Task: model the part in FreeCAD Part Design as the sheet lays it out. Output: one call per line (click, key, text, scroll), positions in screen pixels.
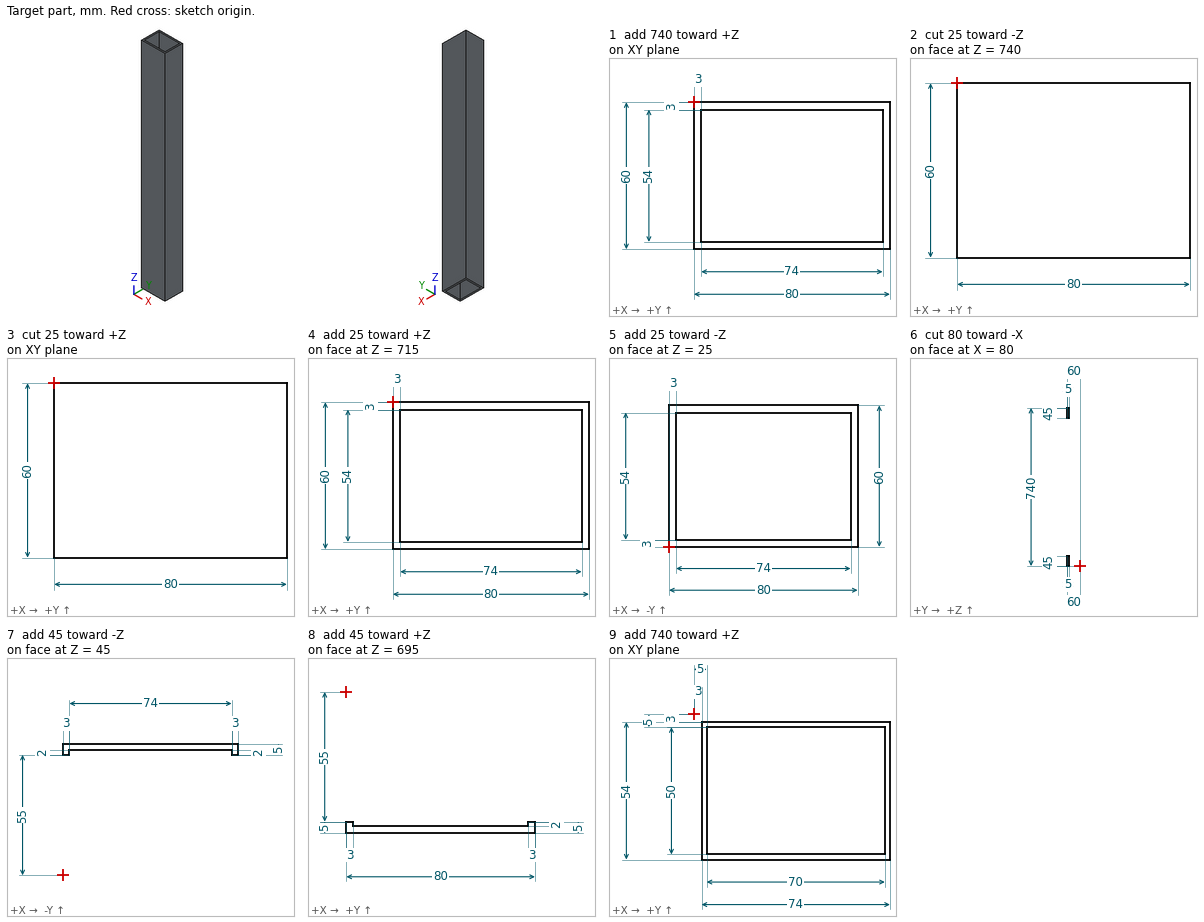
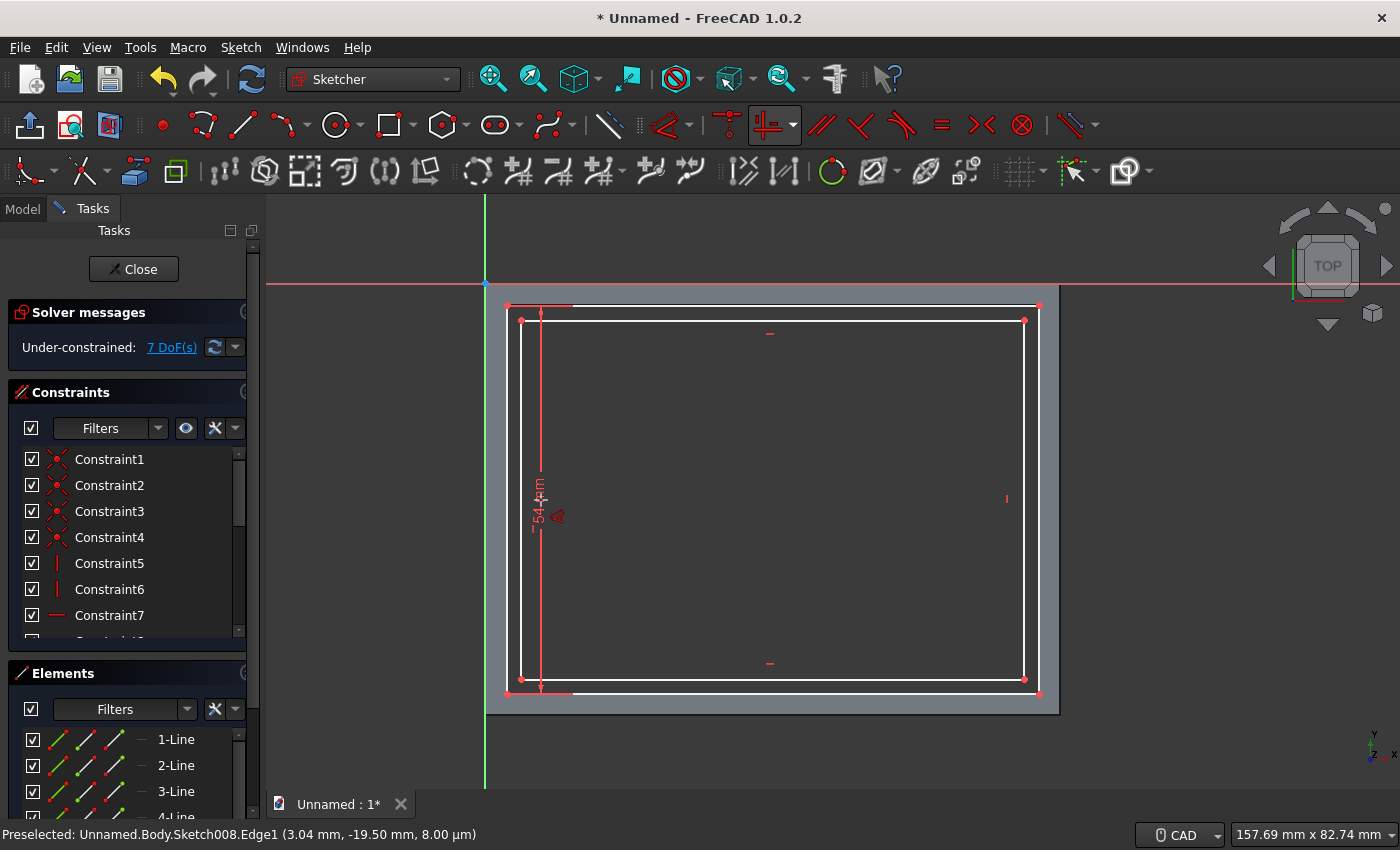
click(667, 694)
click(773, 728)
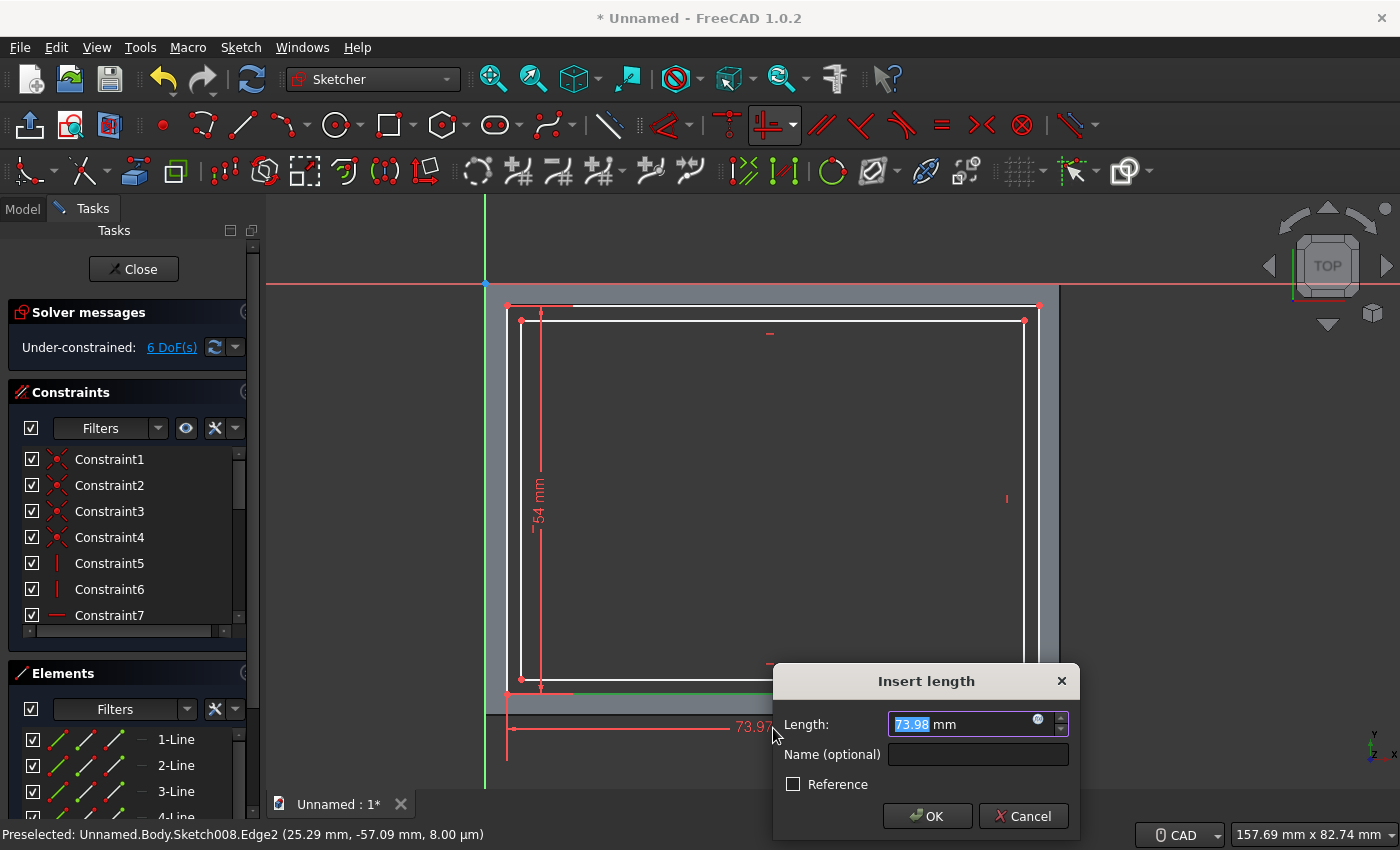
text(74)
key(Return)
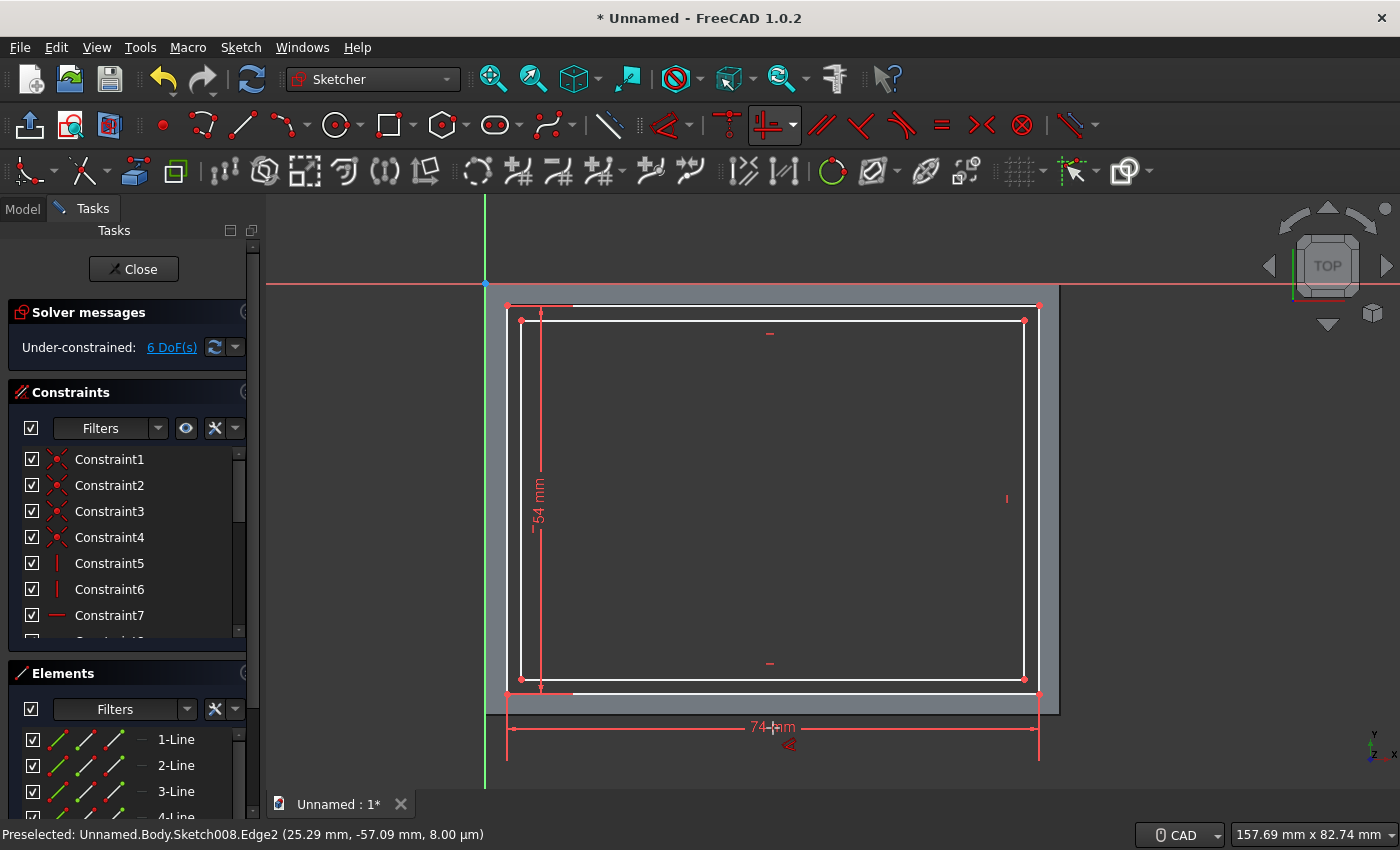
click(521, 429)
click(555, 418)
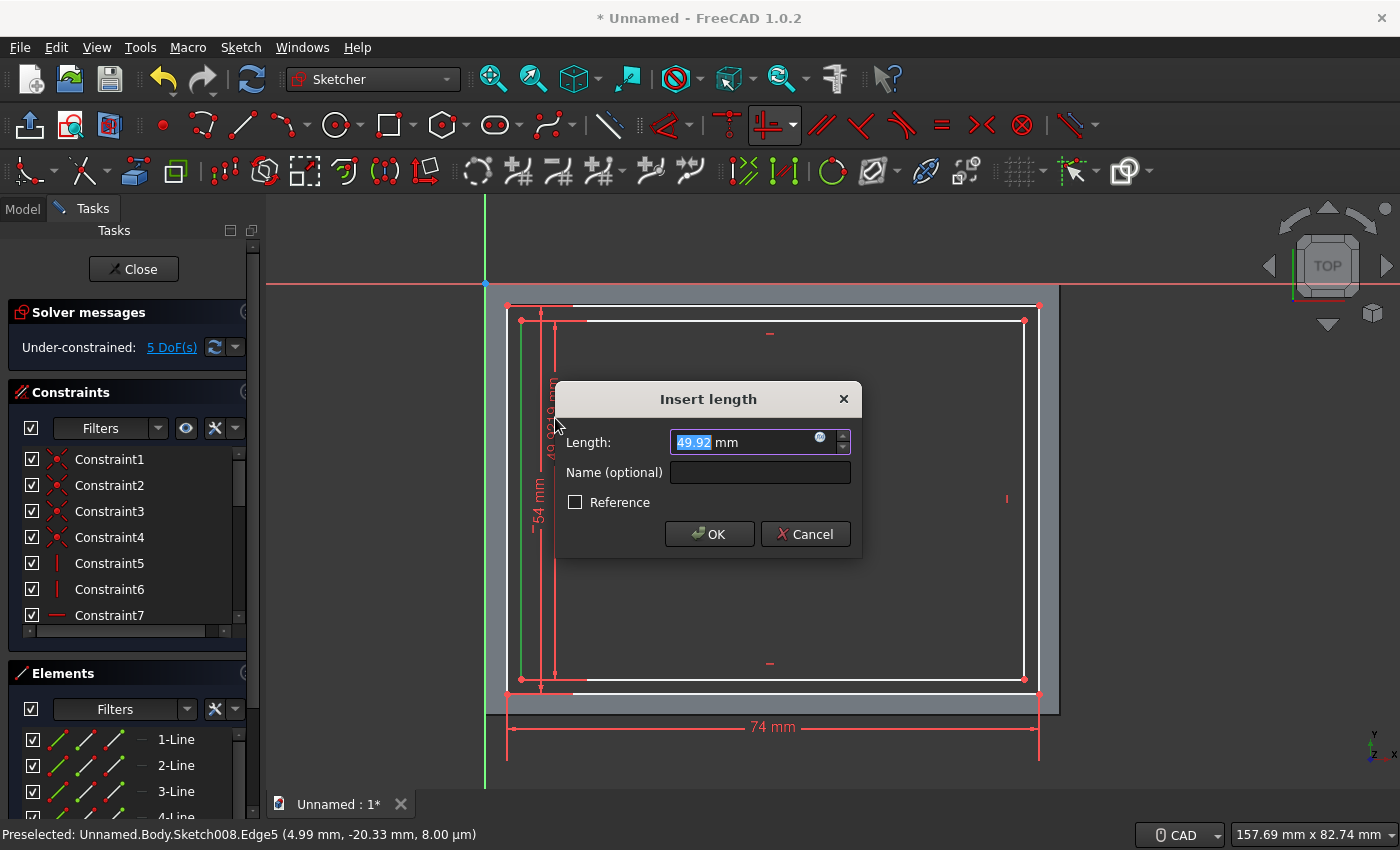
text(50)
key(Return)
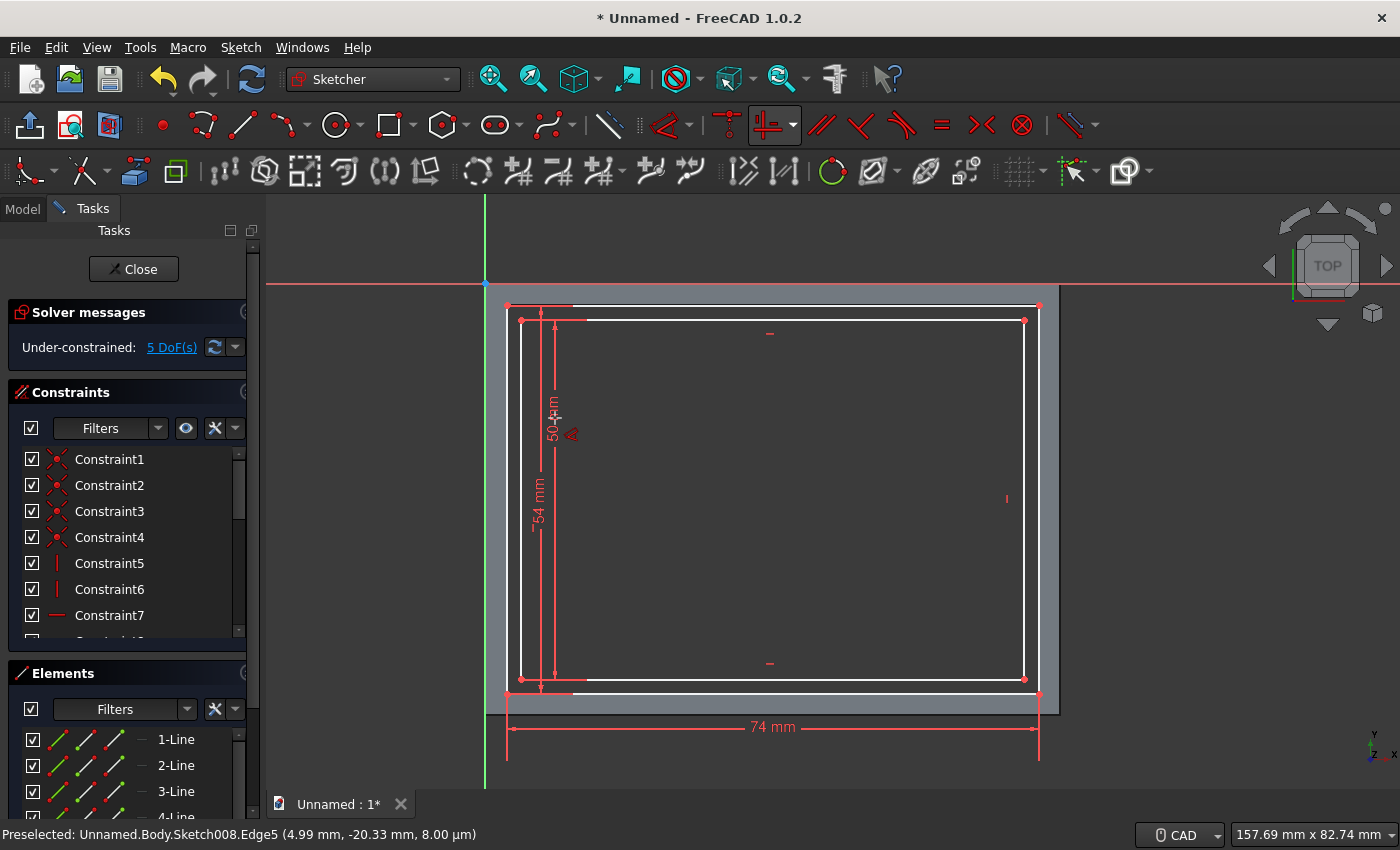
click(672, 680)
click(657, 714)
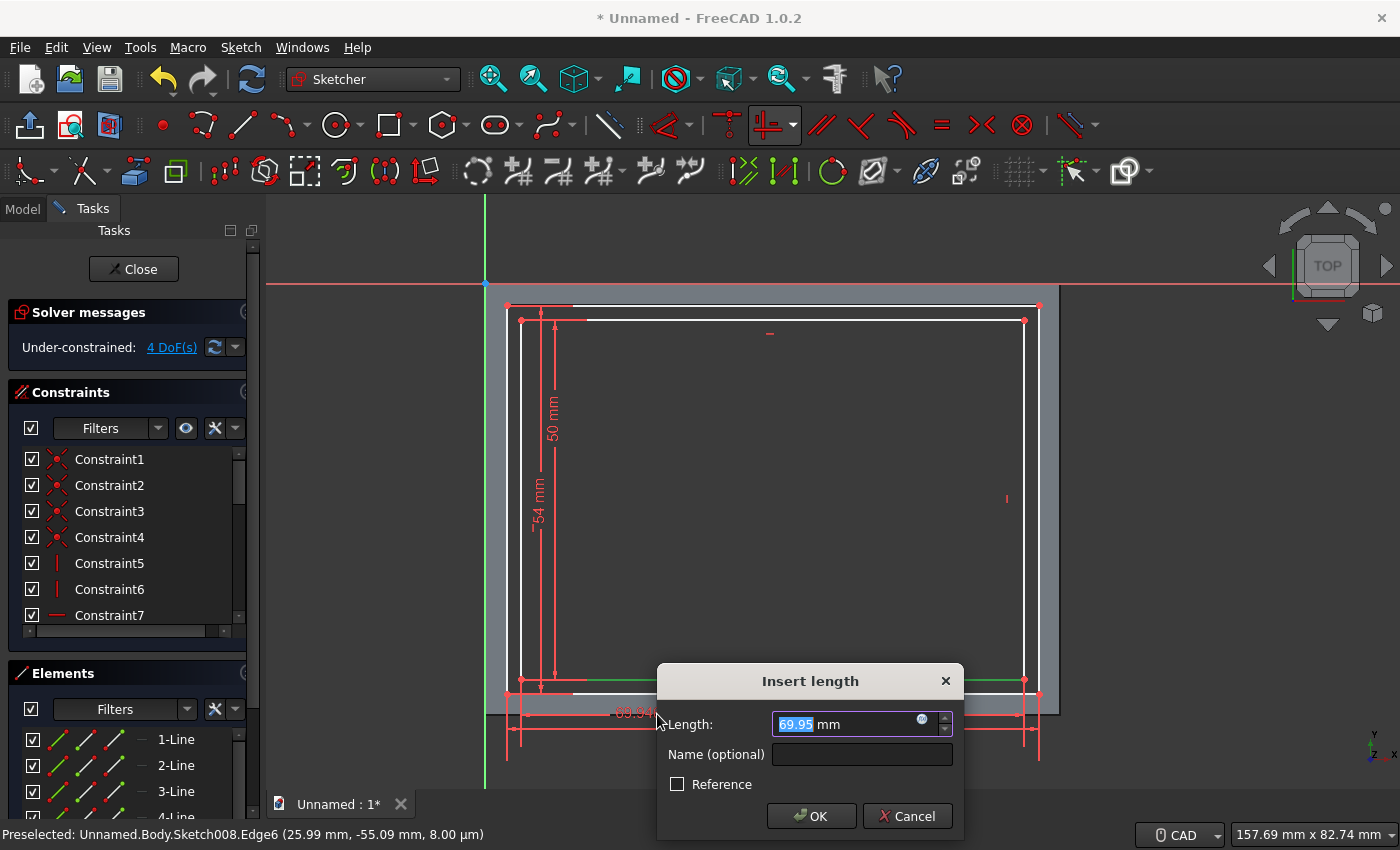
text(70)
key(Return)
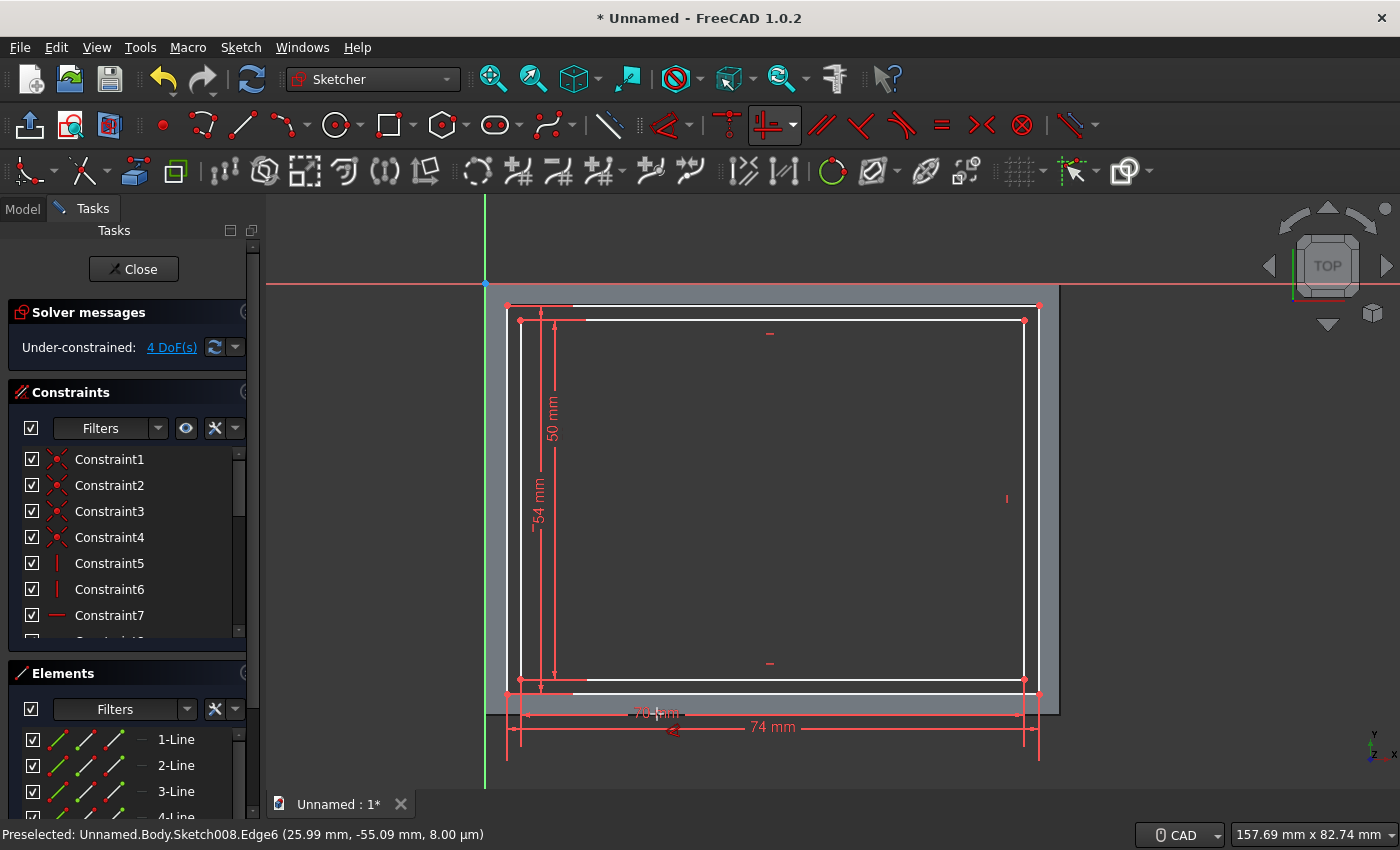
scroll(507, 306, up, 4)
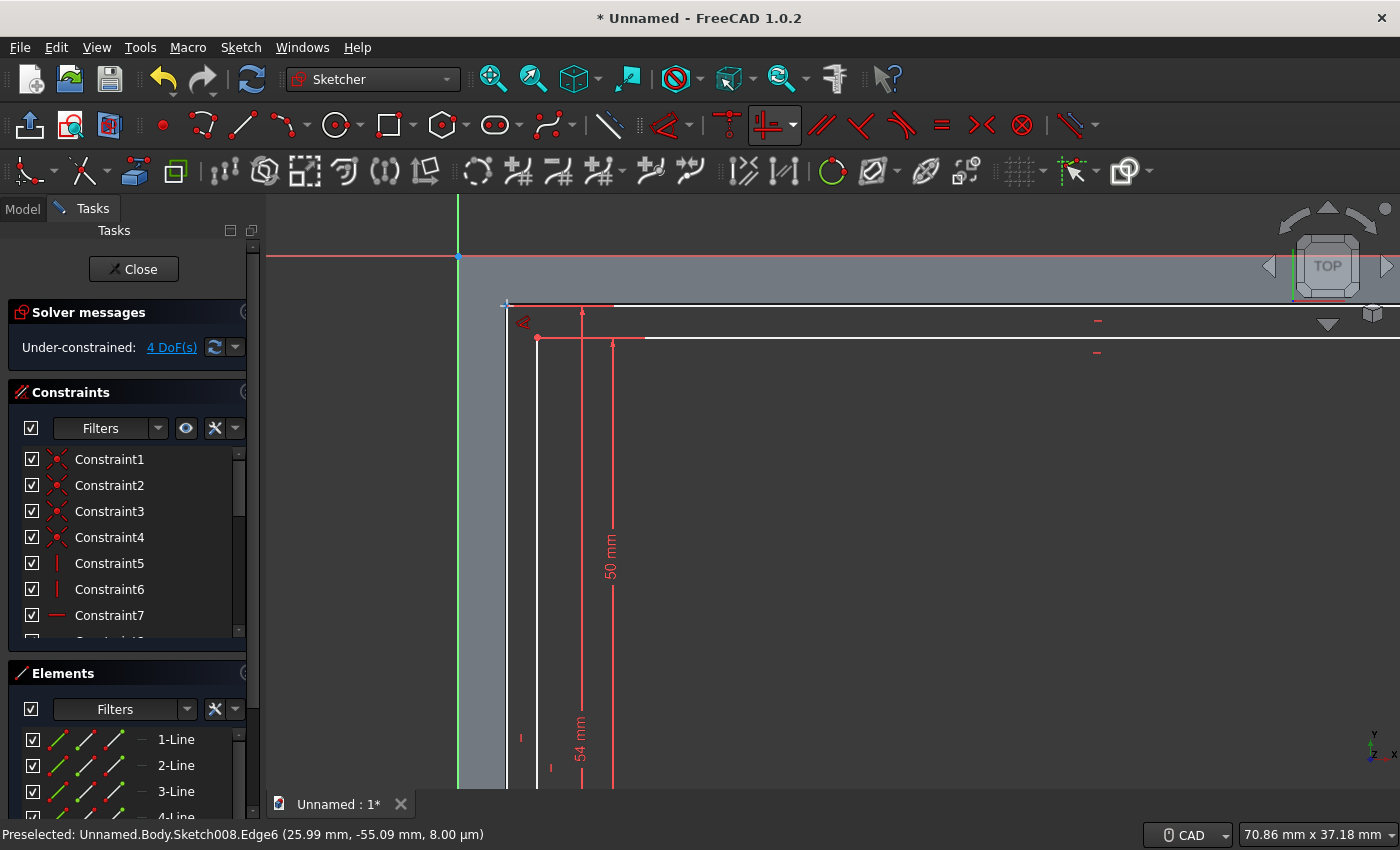
click(507, 306)
click(482, 222)